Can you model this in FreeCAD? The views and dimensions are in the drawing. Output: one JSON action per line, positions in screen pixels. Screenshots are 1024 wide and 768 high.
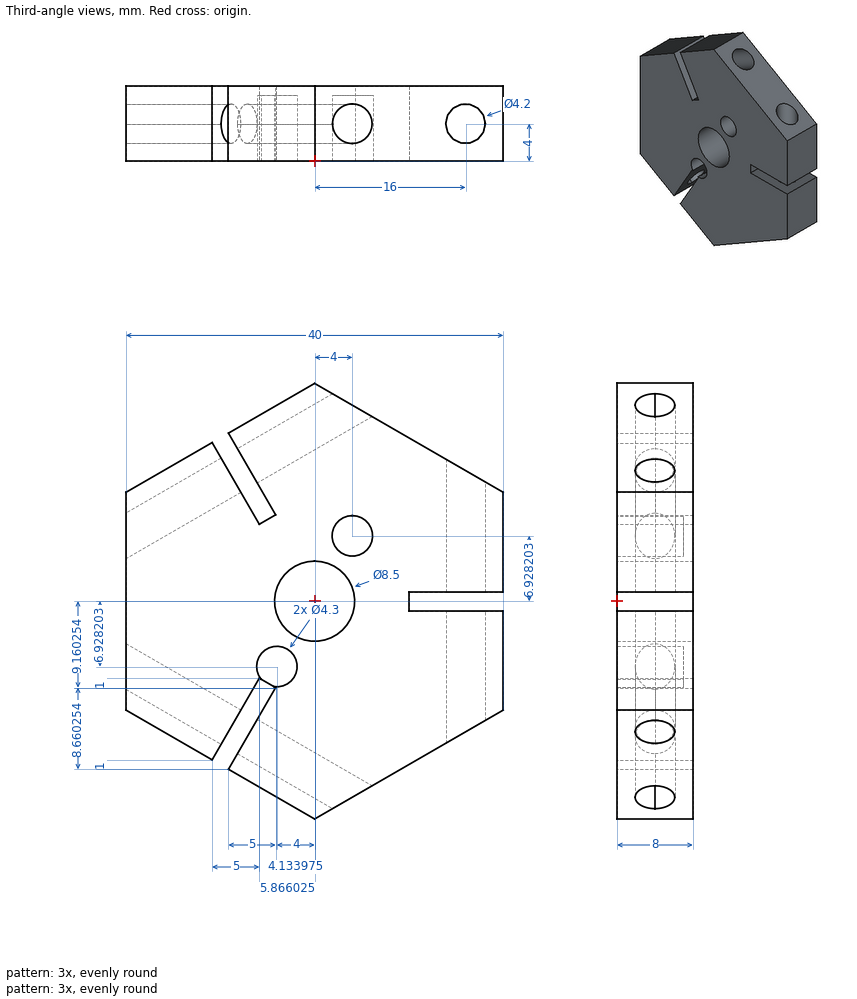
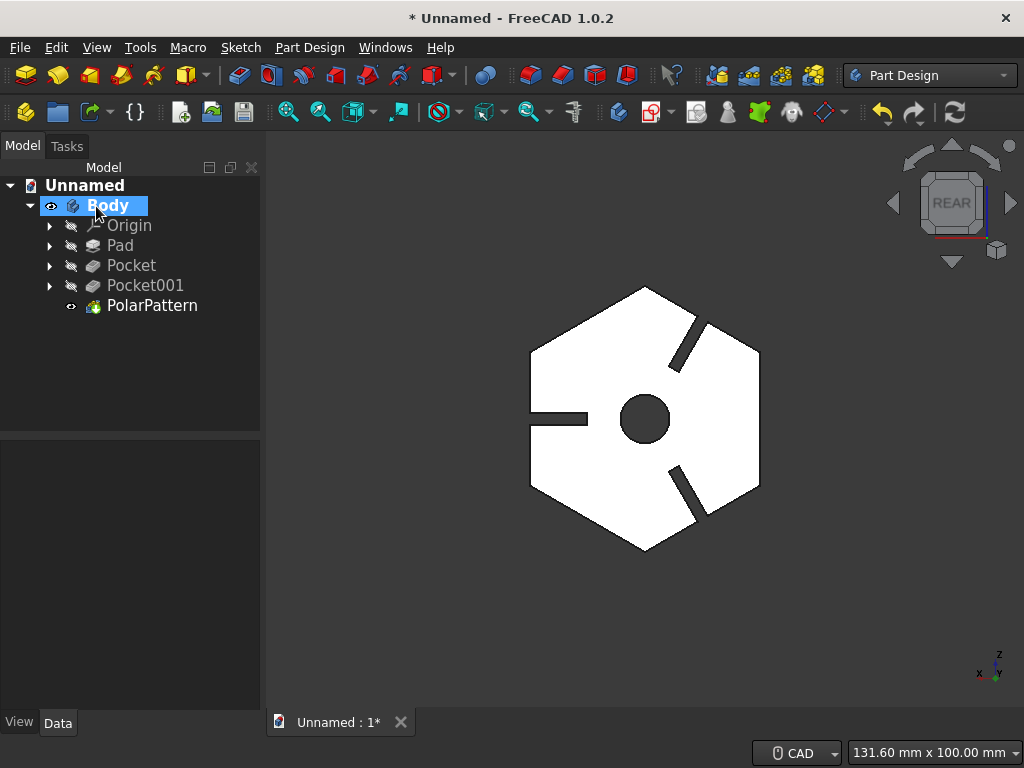
{"action": "left_click", "coordinate": [50, 226]}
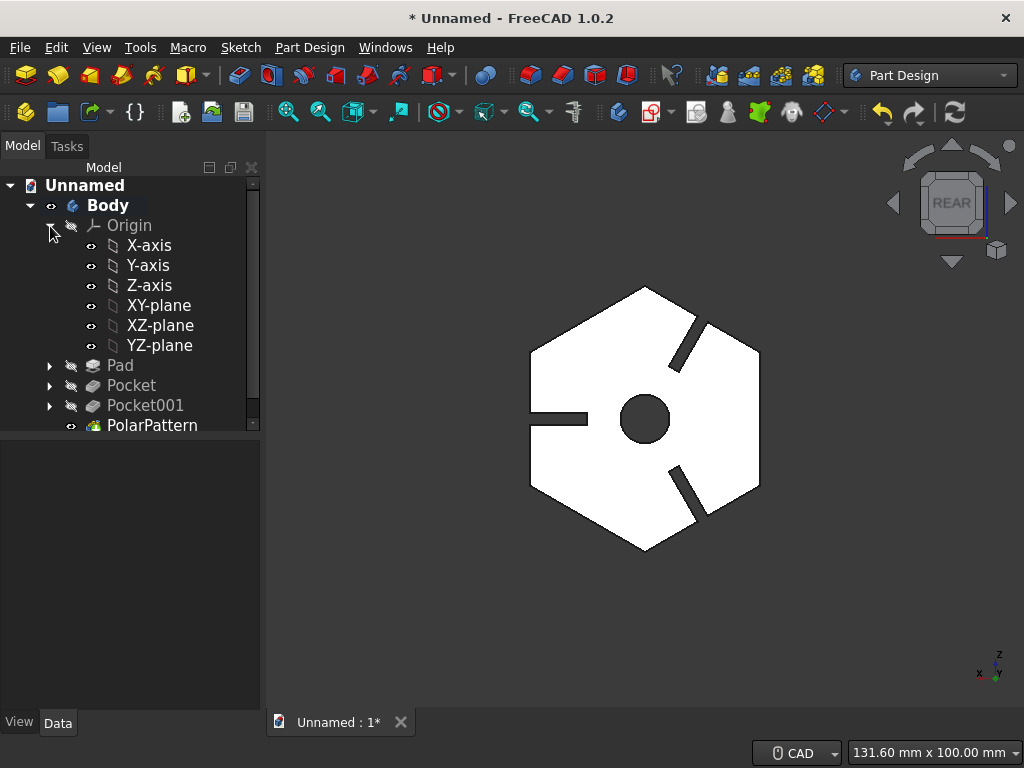
{"action": "left_click", "coordinate": [136, 306]}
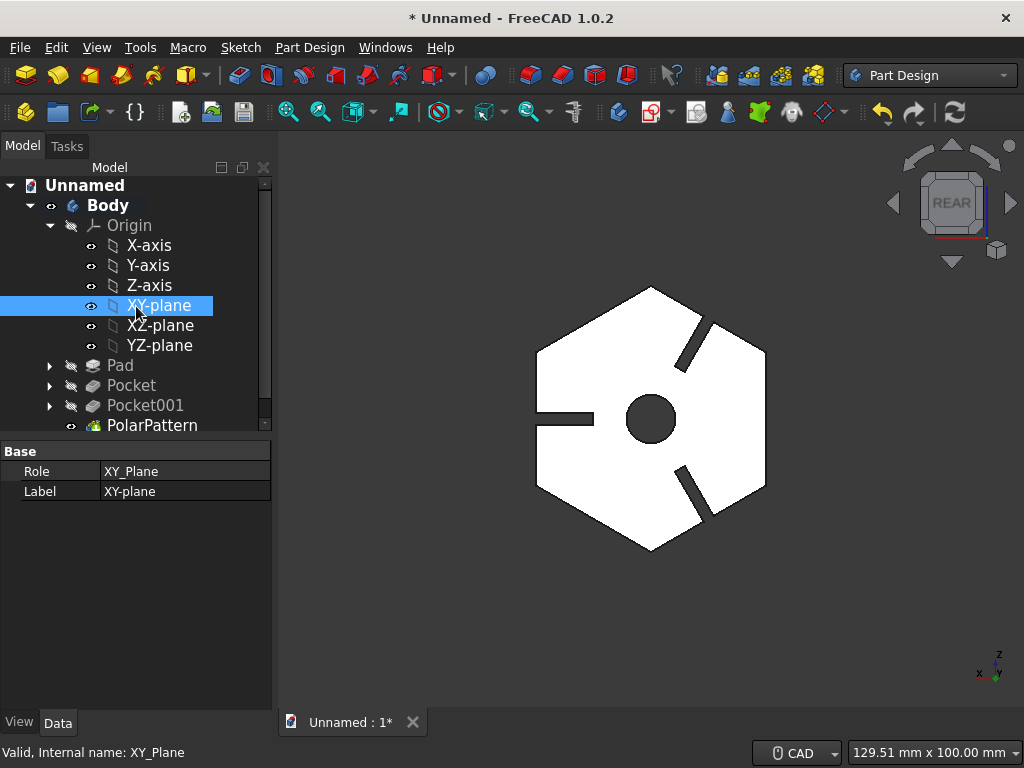
{"action": "left_click", "coordinate": [824, 112]}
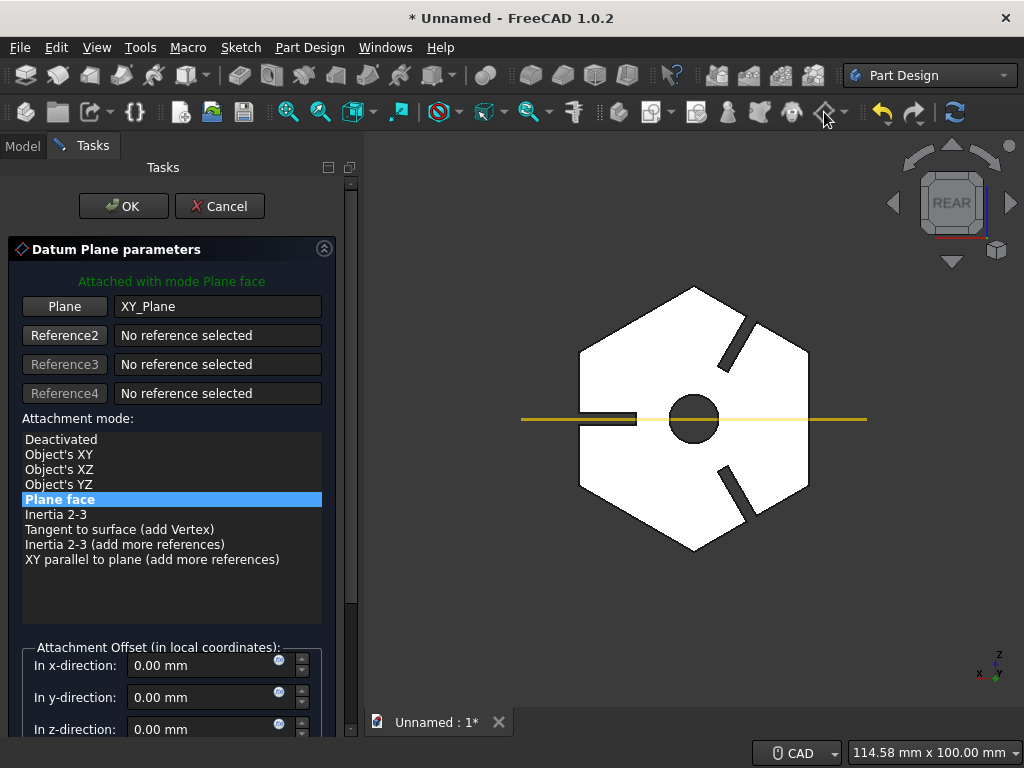
{"action": "scroll", "coordinate": [351, 456], "scroll_direction": "down", "scroll_amount": 2}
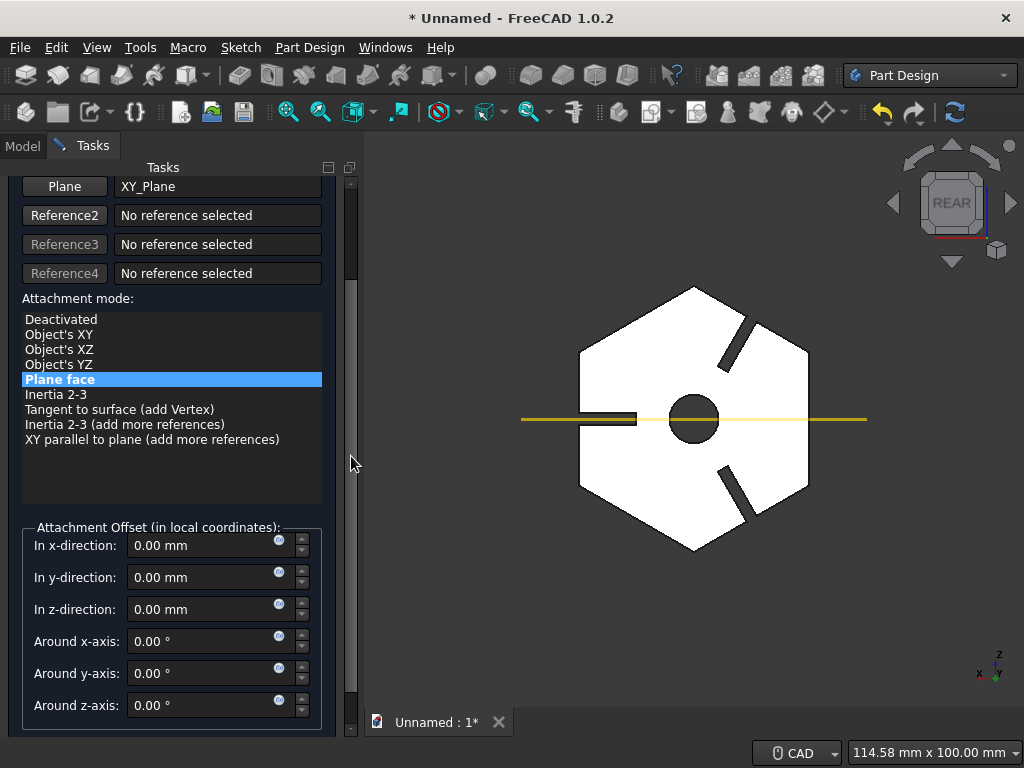
{"action": "triple_click", "coordinate": [210, 609]}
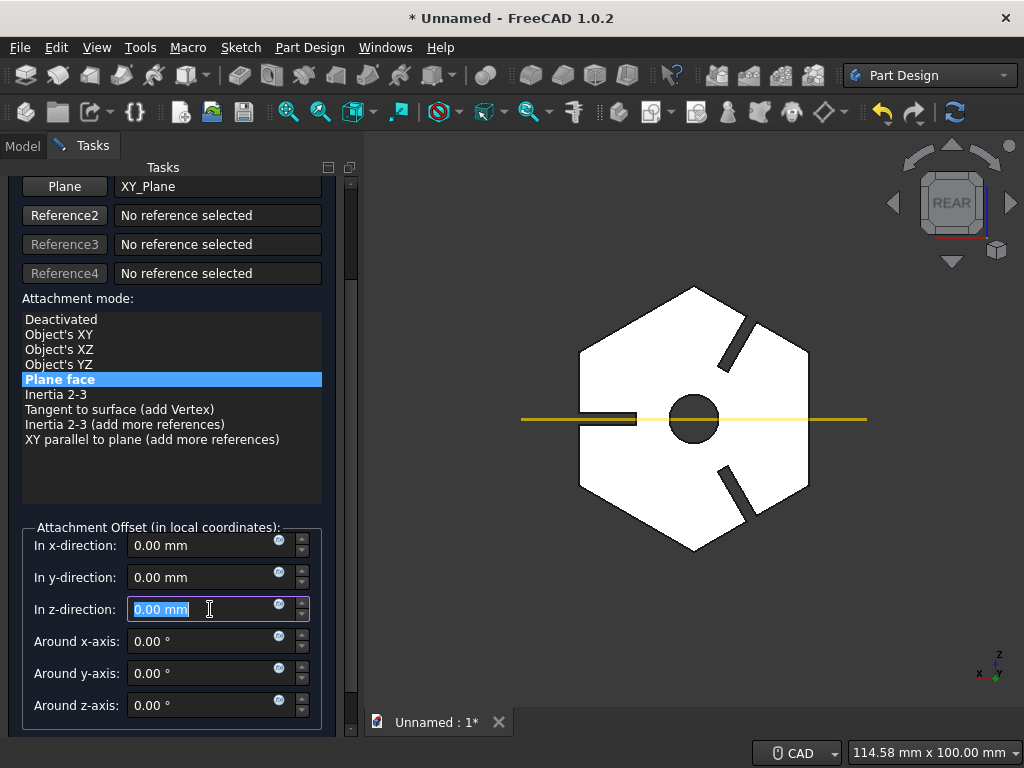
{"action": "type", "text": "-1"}
{"action": "key", "text": "Tab"}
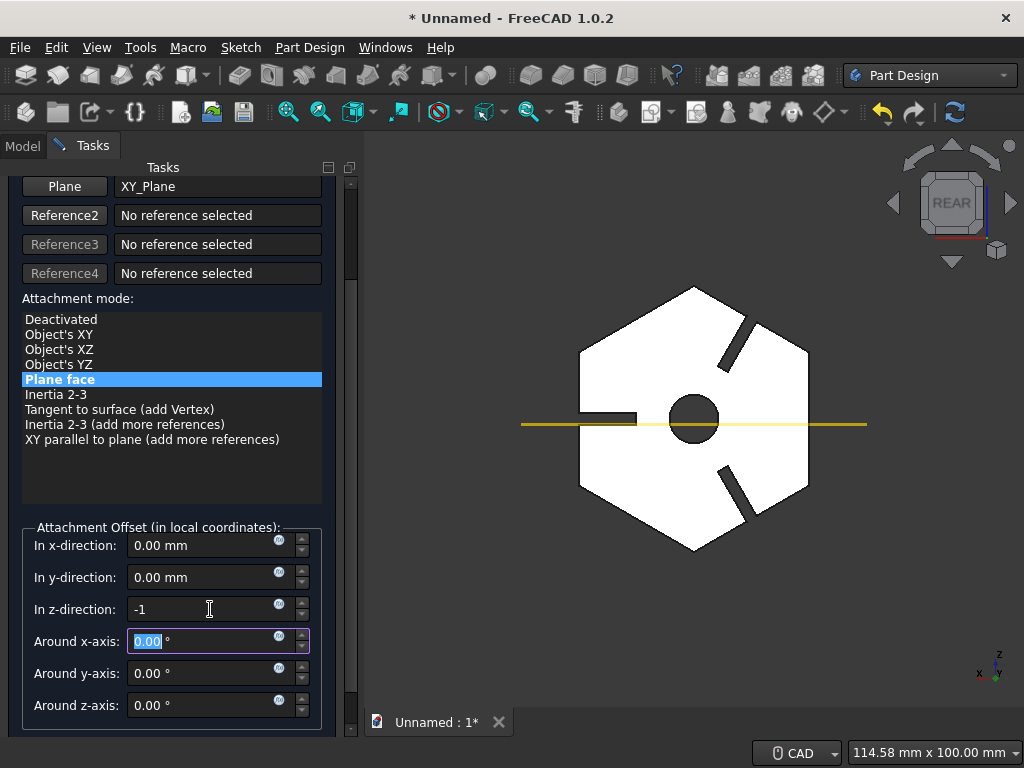
{"action": "scroll", "coordinate": [351, 456], "scroll_direction": "up", "scroll_amount": 3}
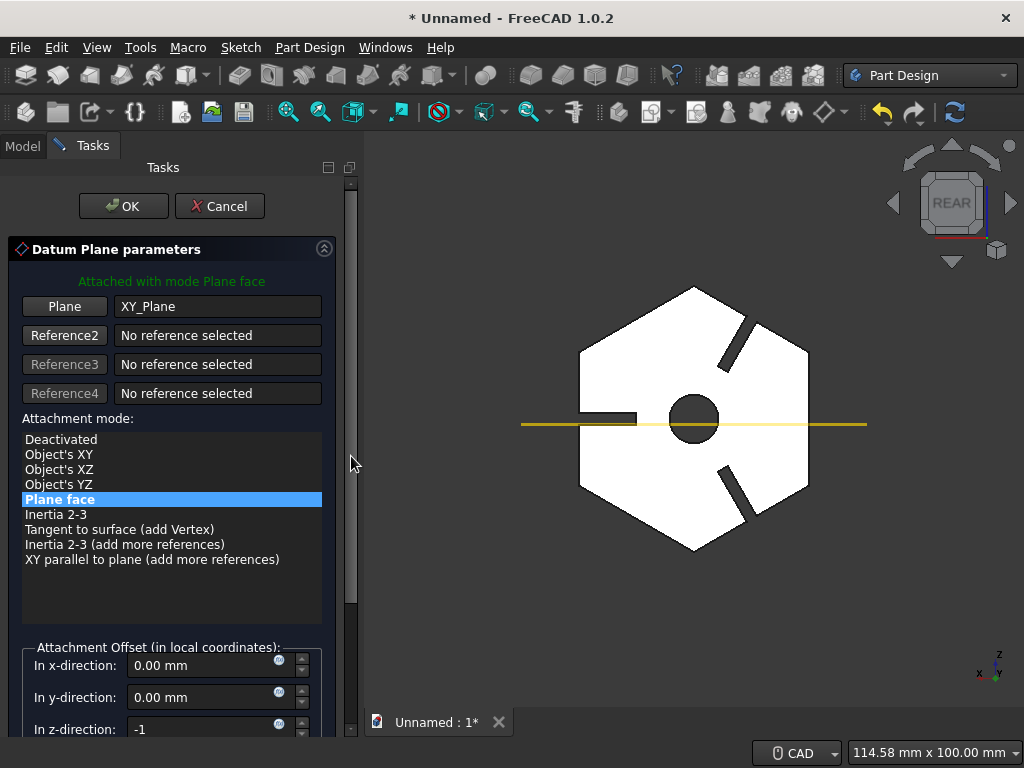
{"action": "left_click", "coordinate": [124, 206]}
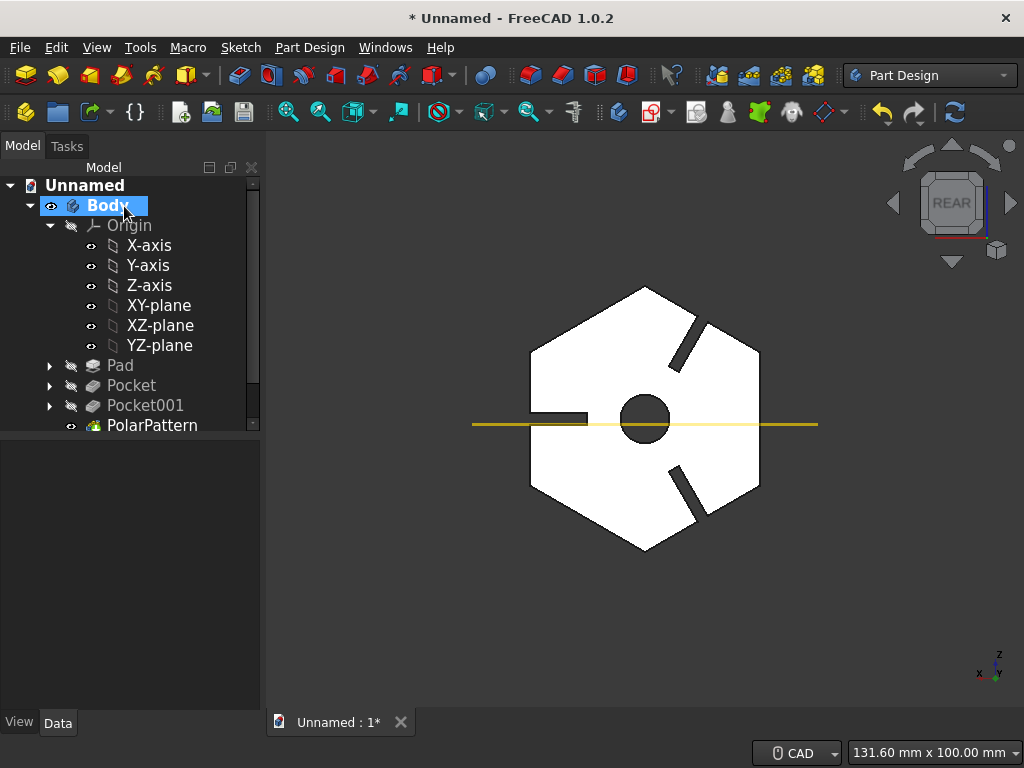
{"action": "scroll", "coordinate": [100, 301], "scroll_direction": "down", "scroll_amount": 3}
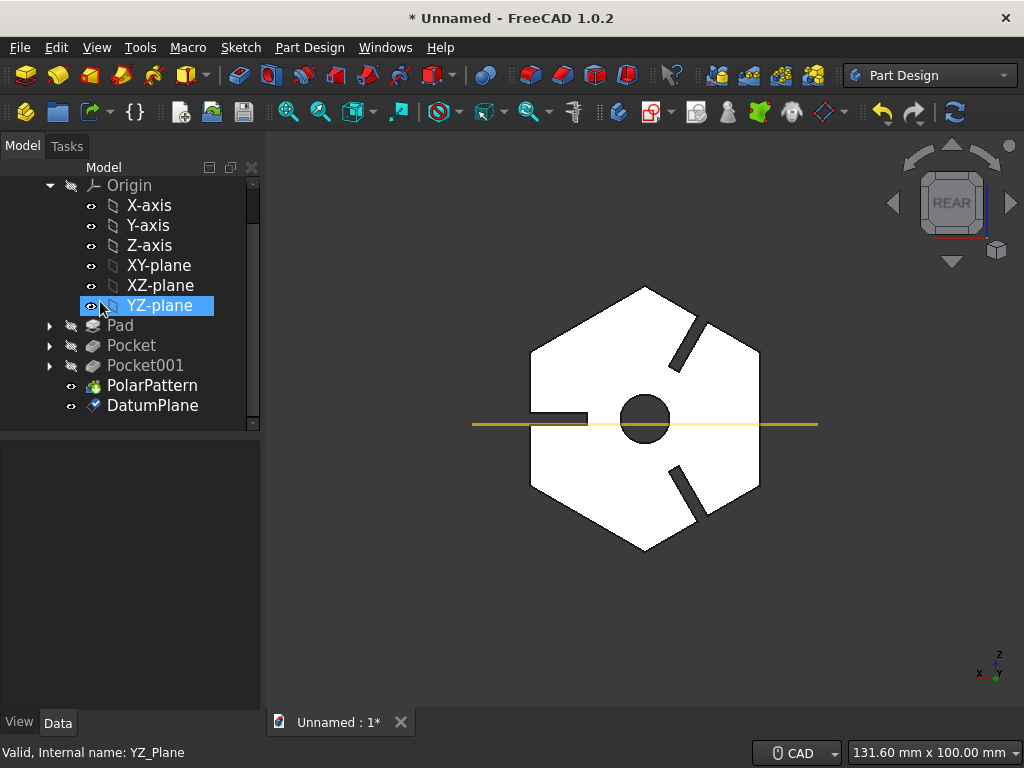
{"action": "left_click", "coordinate": [116, 406]}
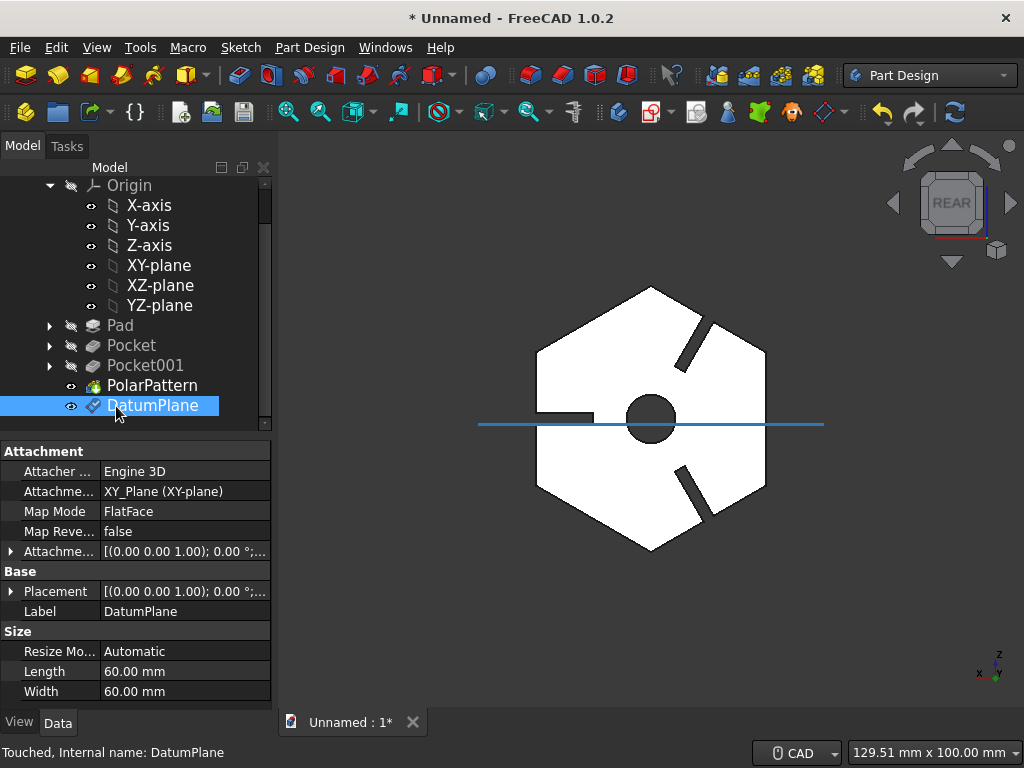
{"action": "left_click", "coordinate": [652, 112]}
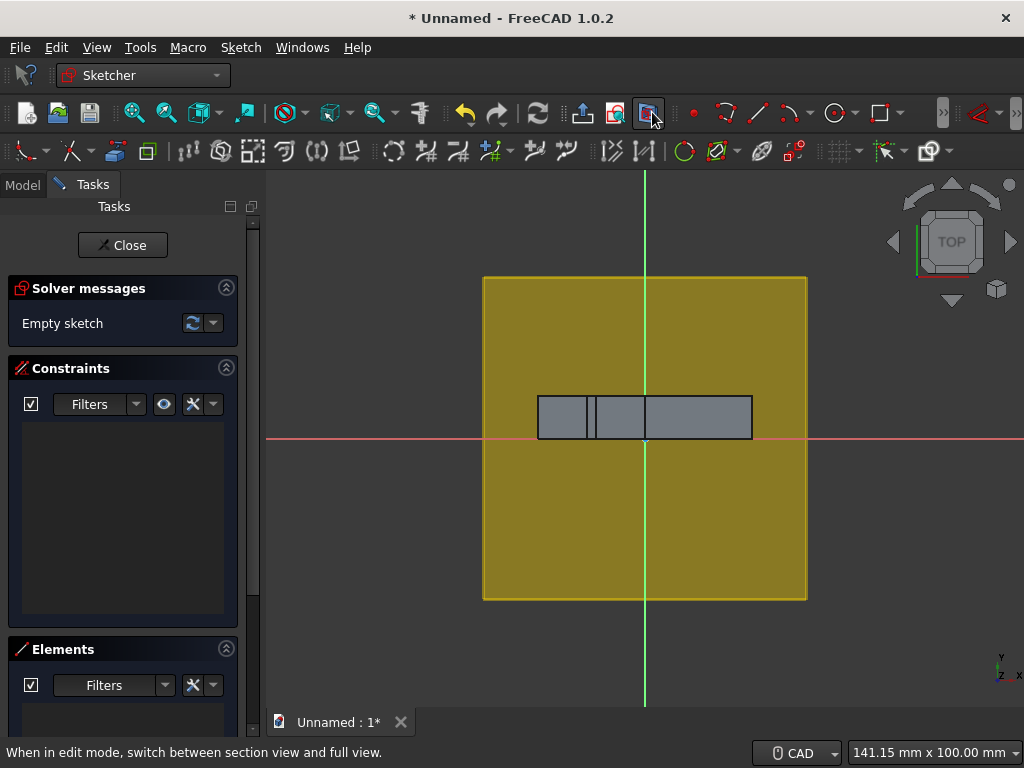
{"action": "left_click", "coordinate": [648, 114]}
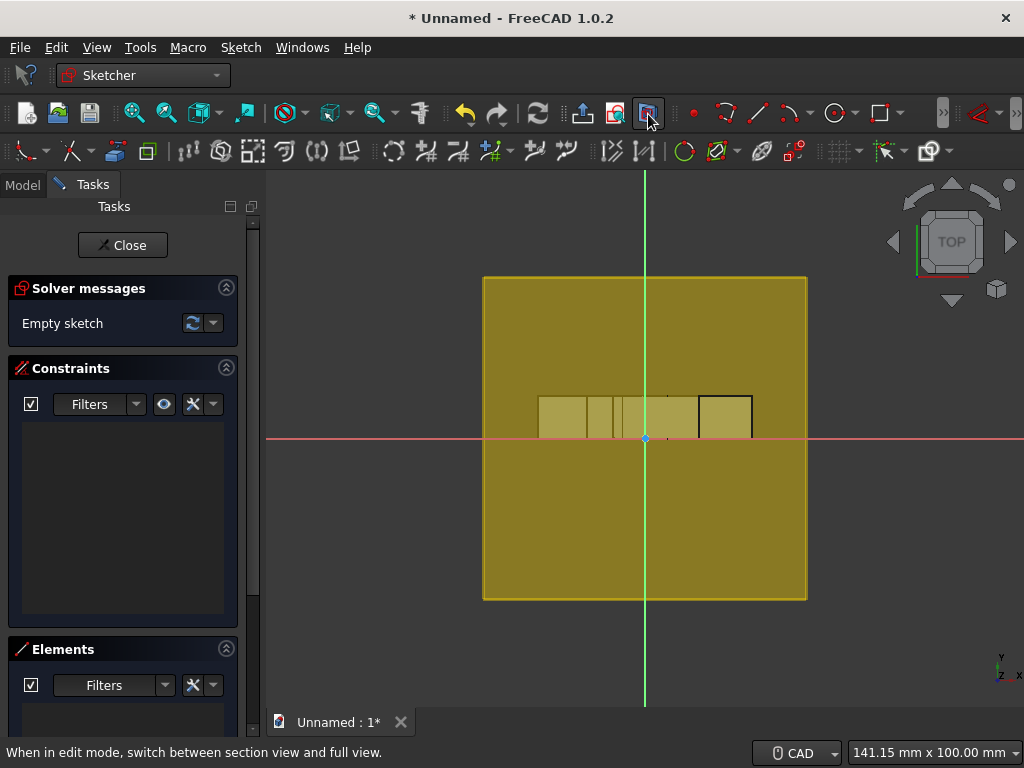
{"action": "scroll", "coordinate": [741, 416], "scroll_direction": "up", "scroll_amount": 14}